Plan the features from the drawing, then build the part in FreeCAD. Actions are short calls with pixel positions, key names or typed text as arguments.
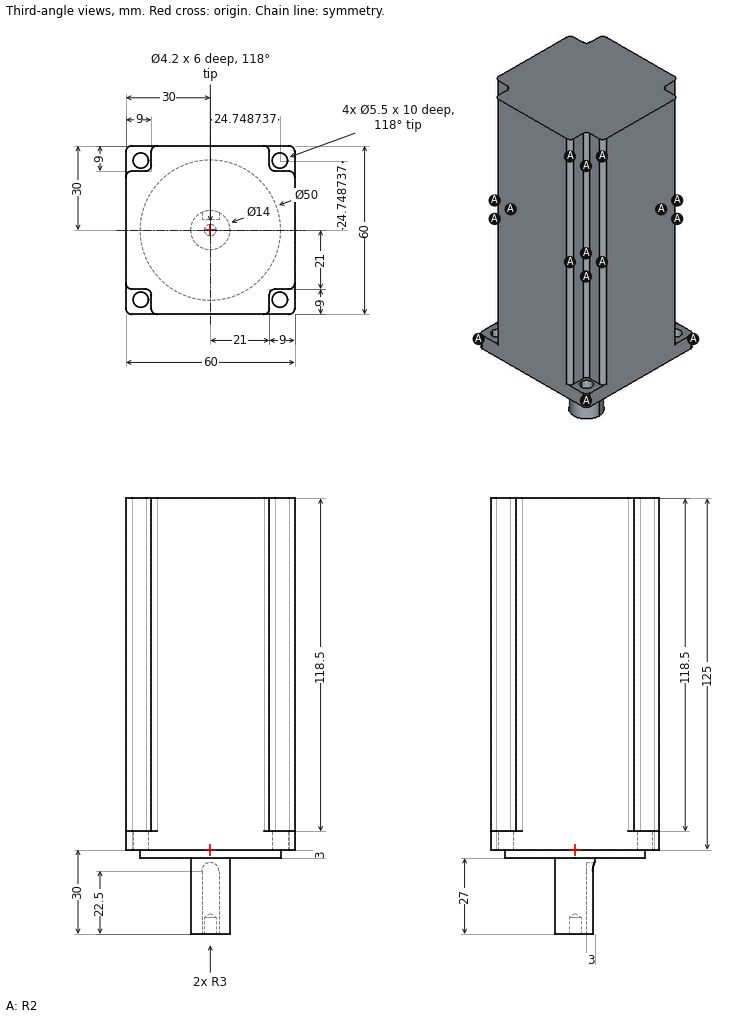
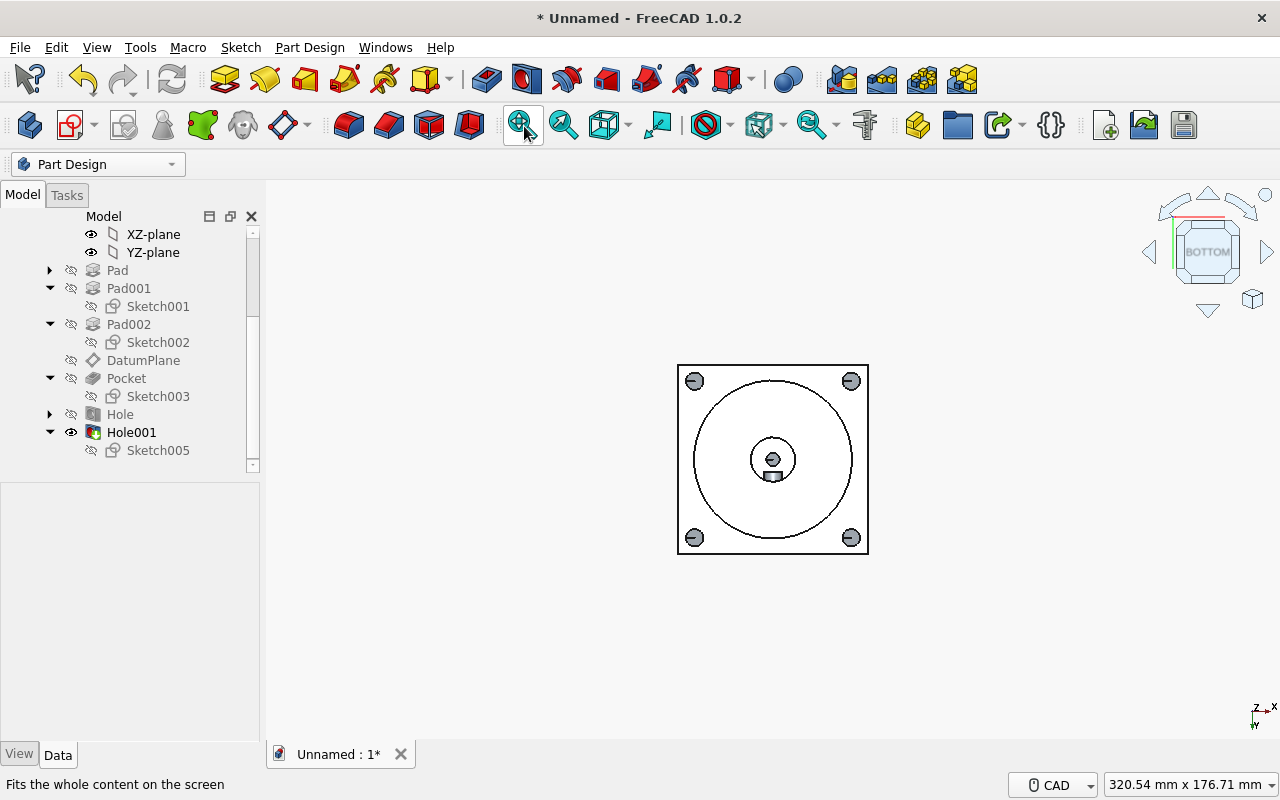
key(0)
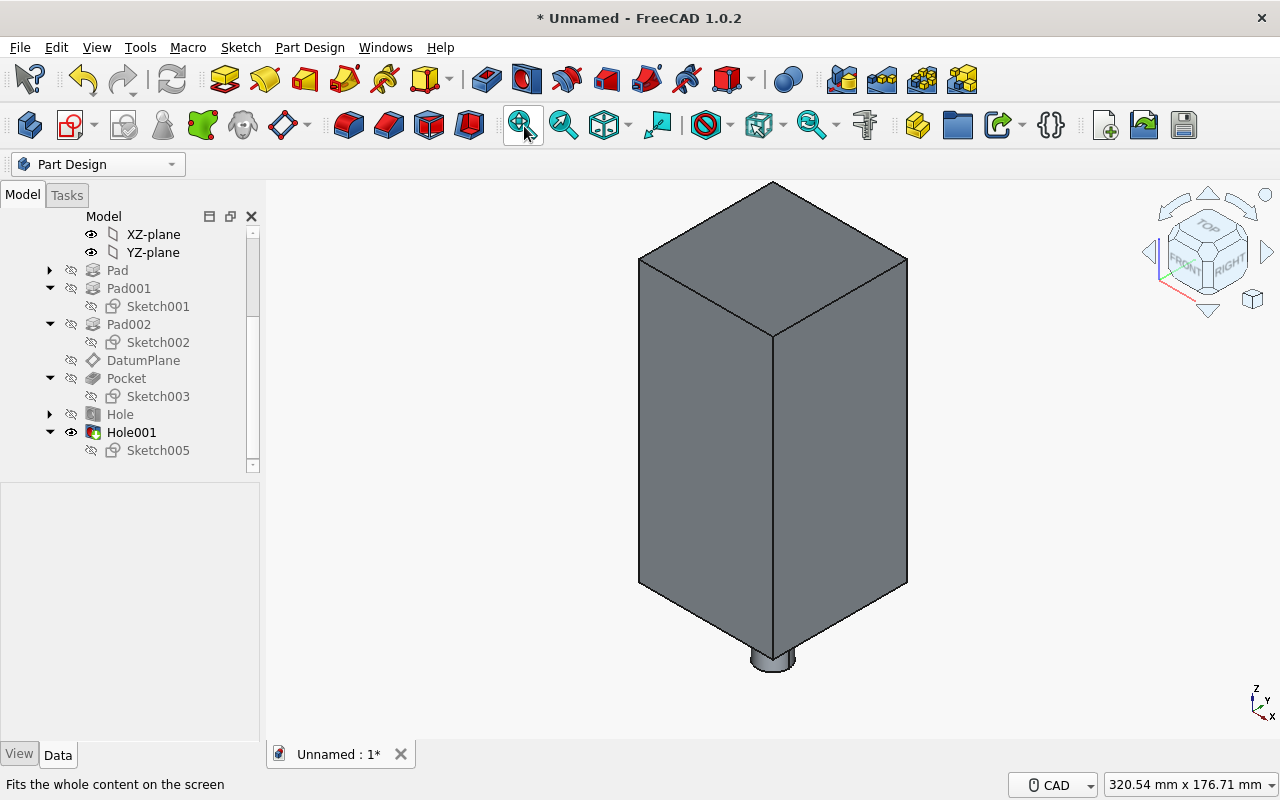
click(773, 258)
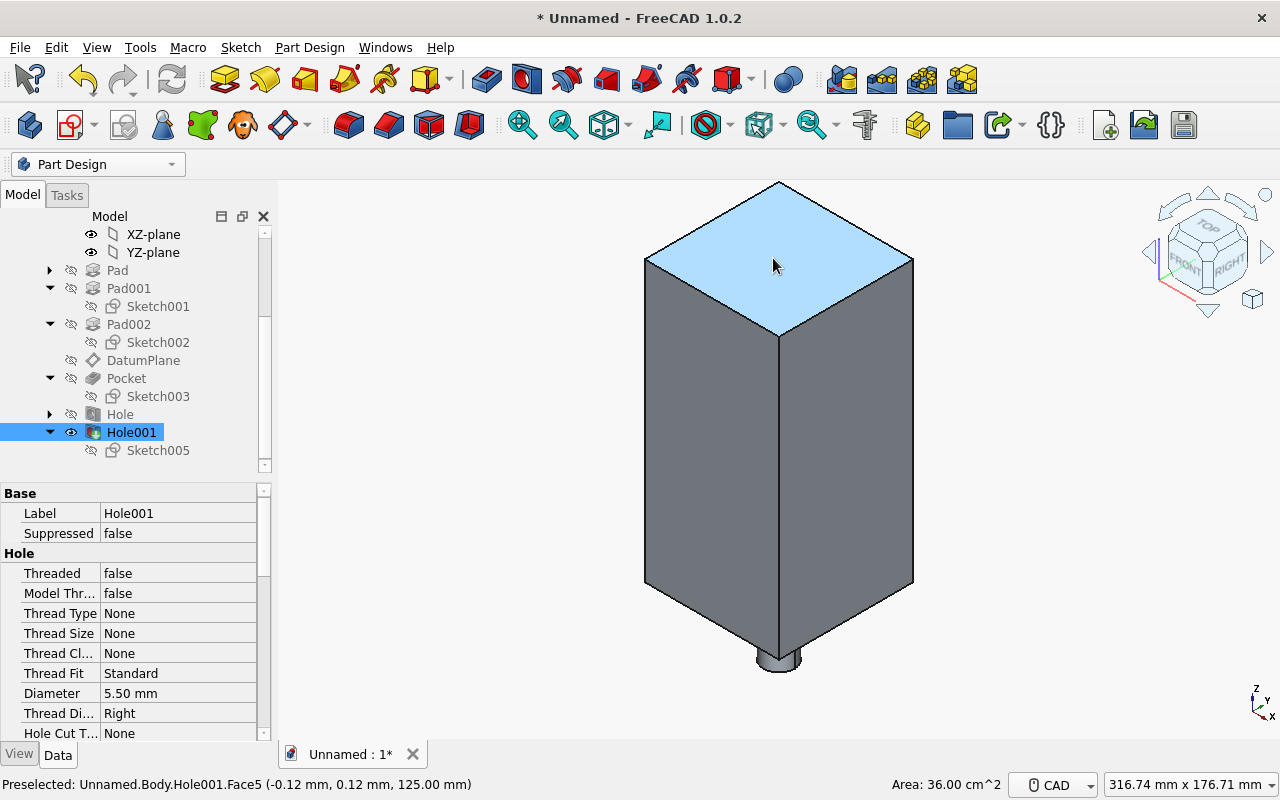
click(70, 126)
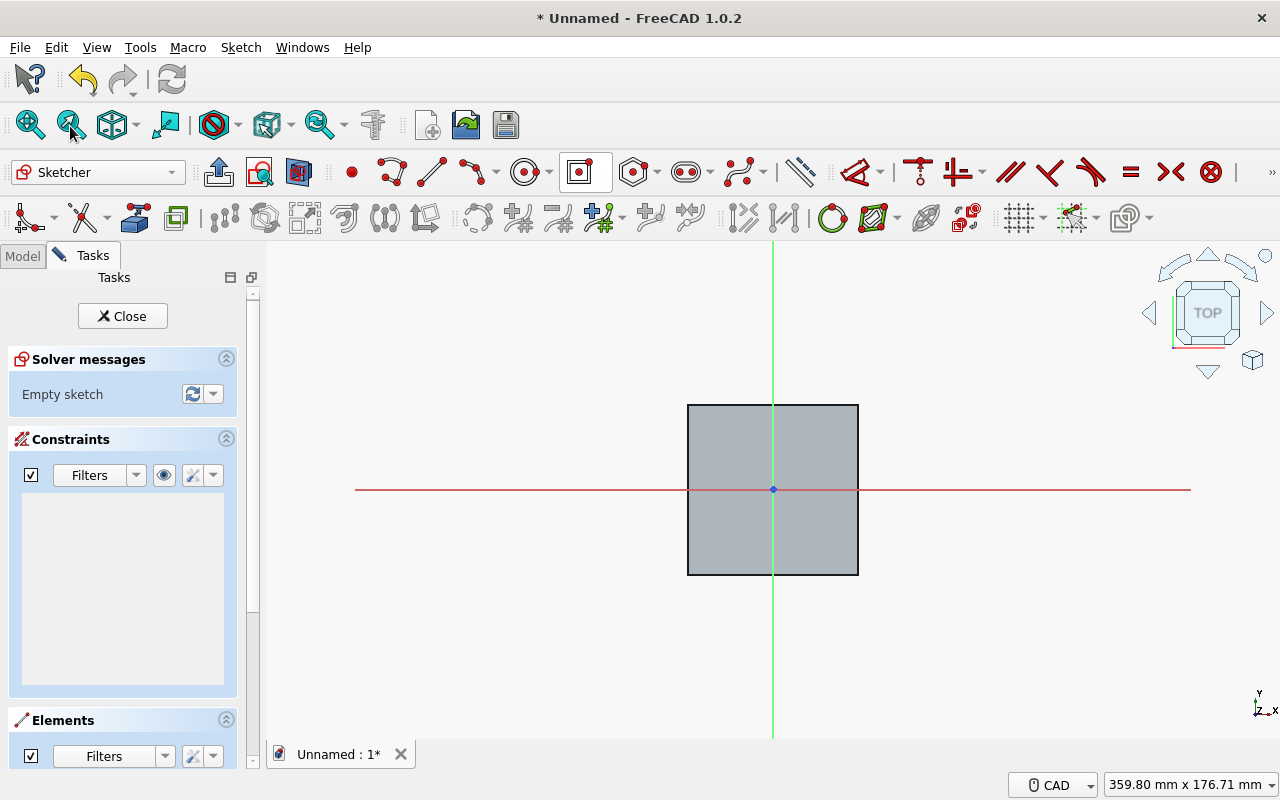
scroll(701, 412, up, 13)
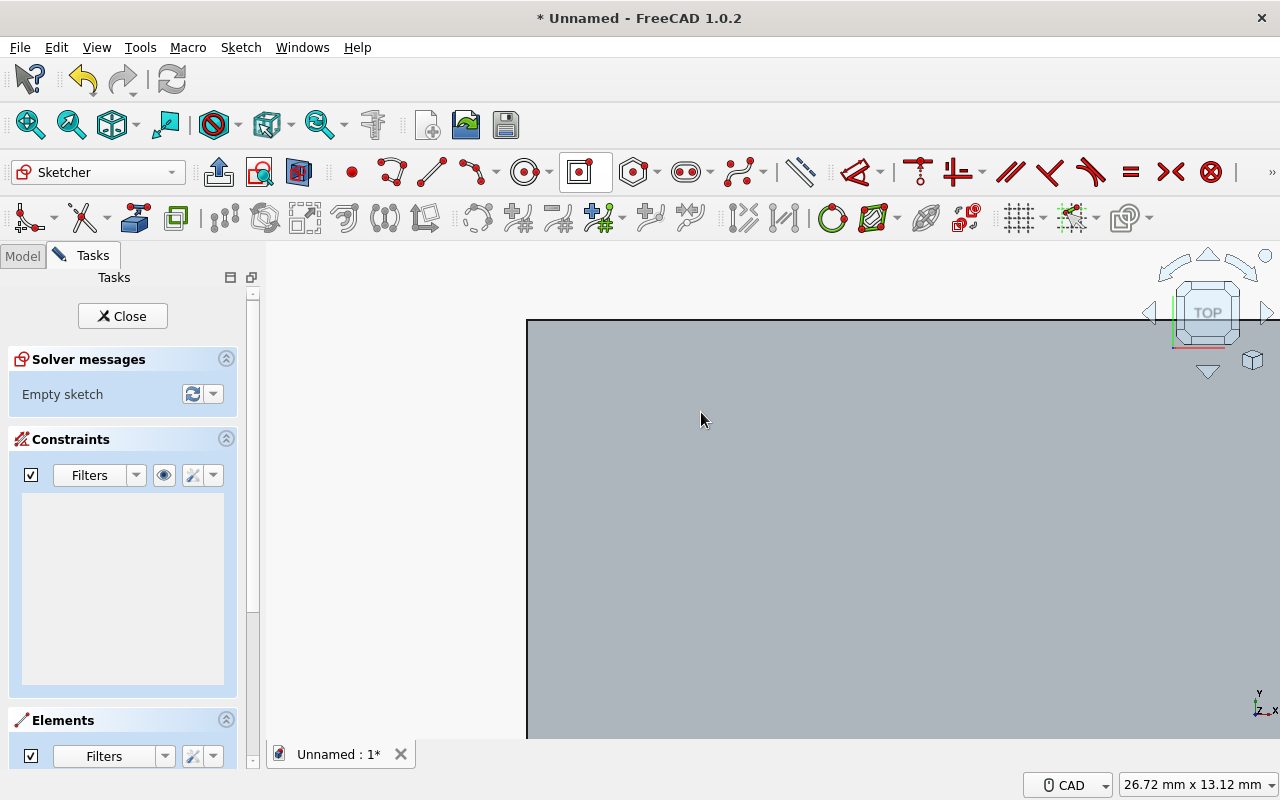
click(606, 172)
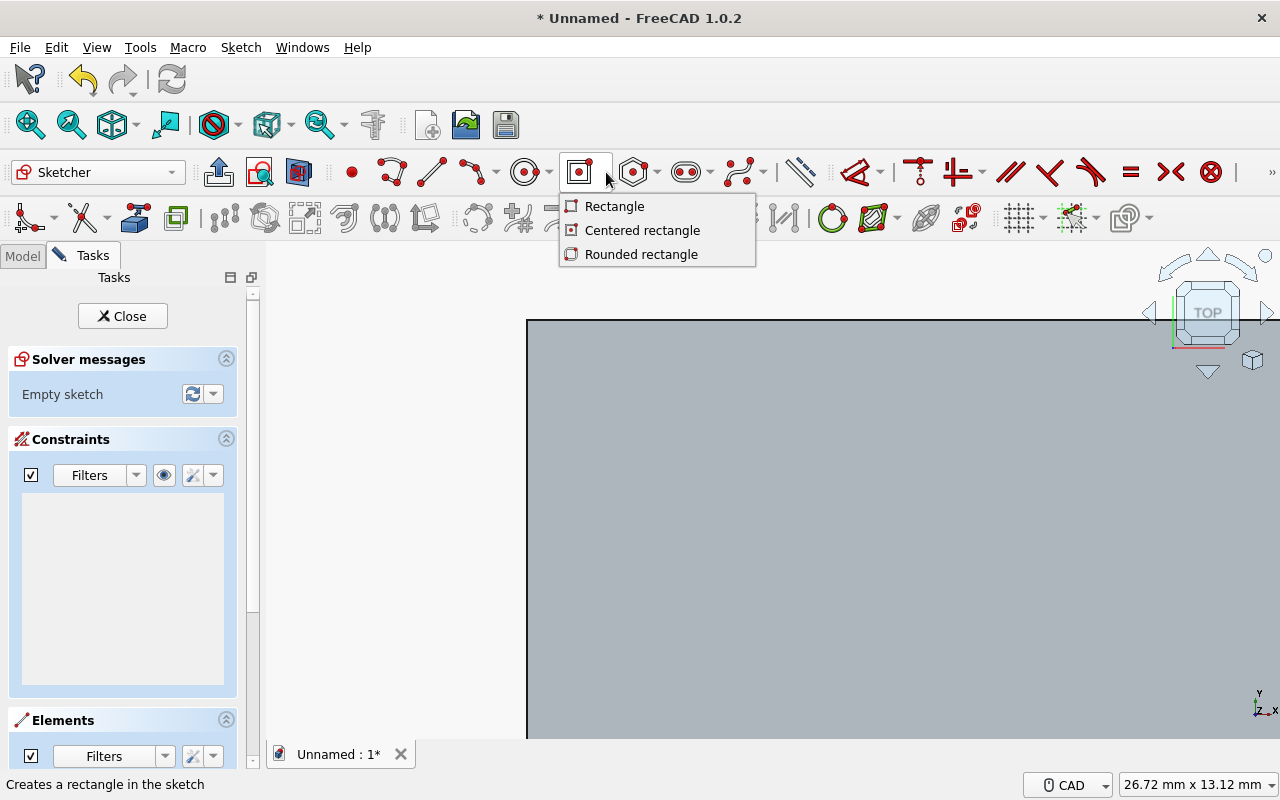
click(658, 206)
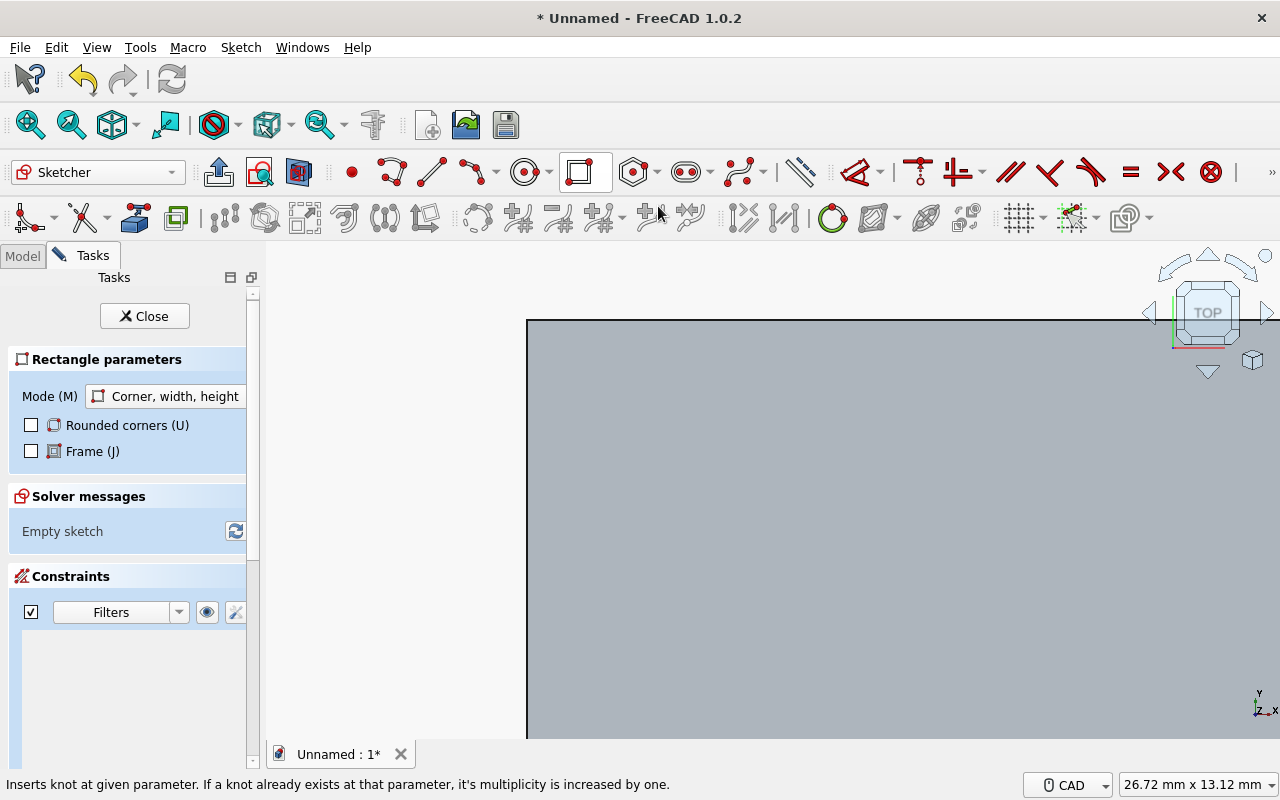
click(527, 320)
move(868, 661)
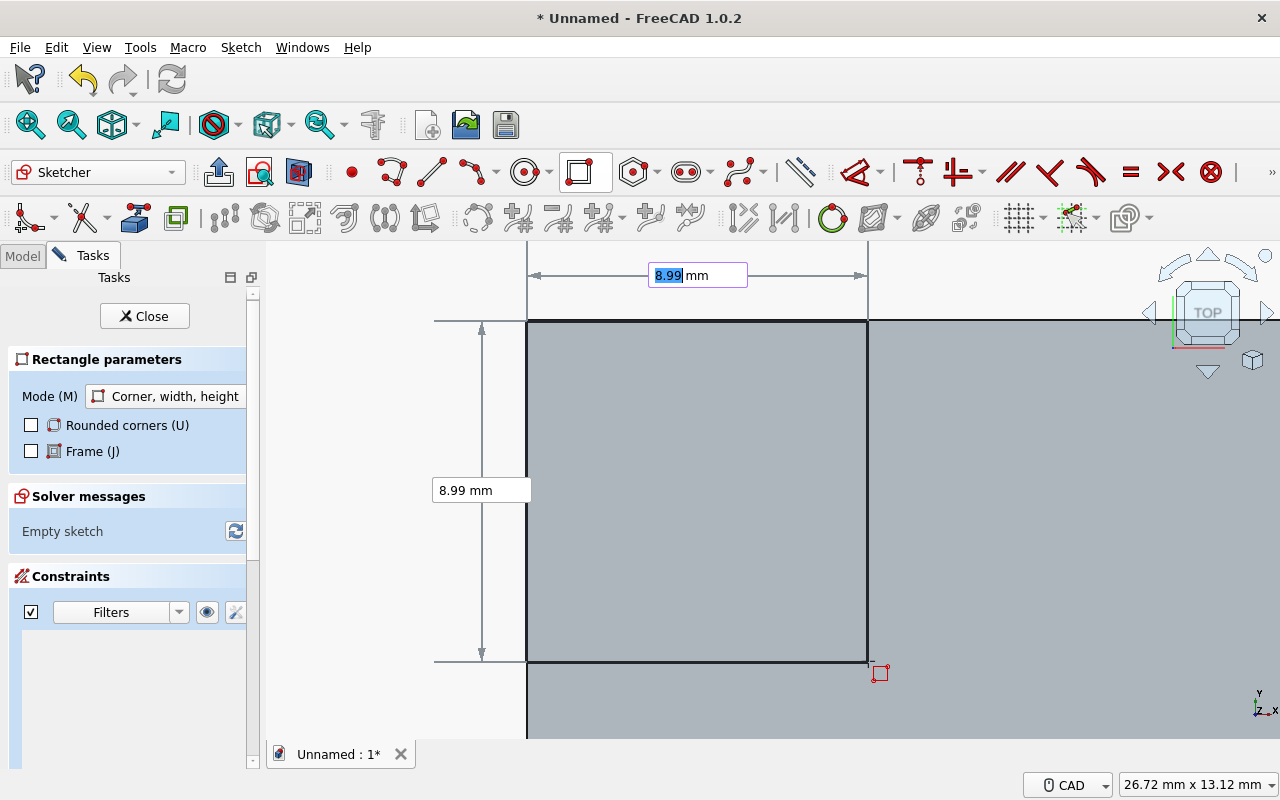
text(9)
key(Tab)
text(9)
key(Return)
key(Escape)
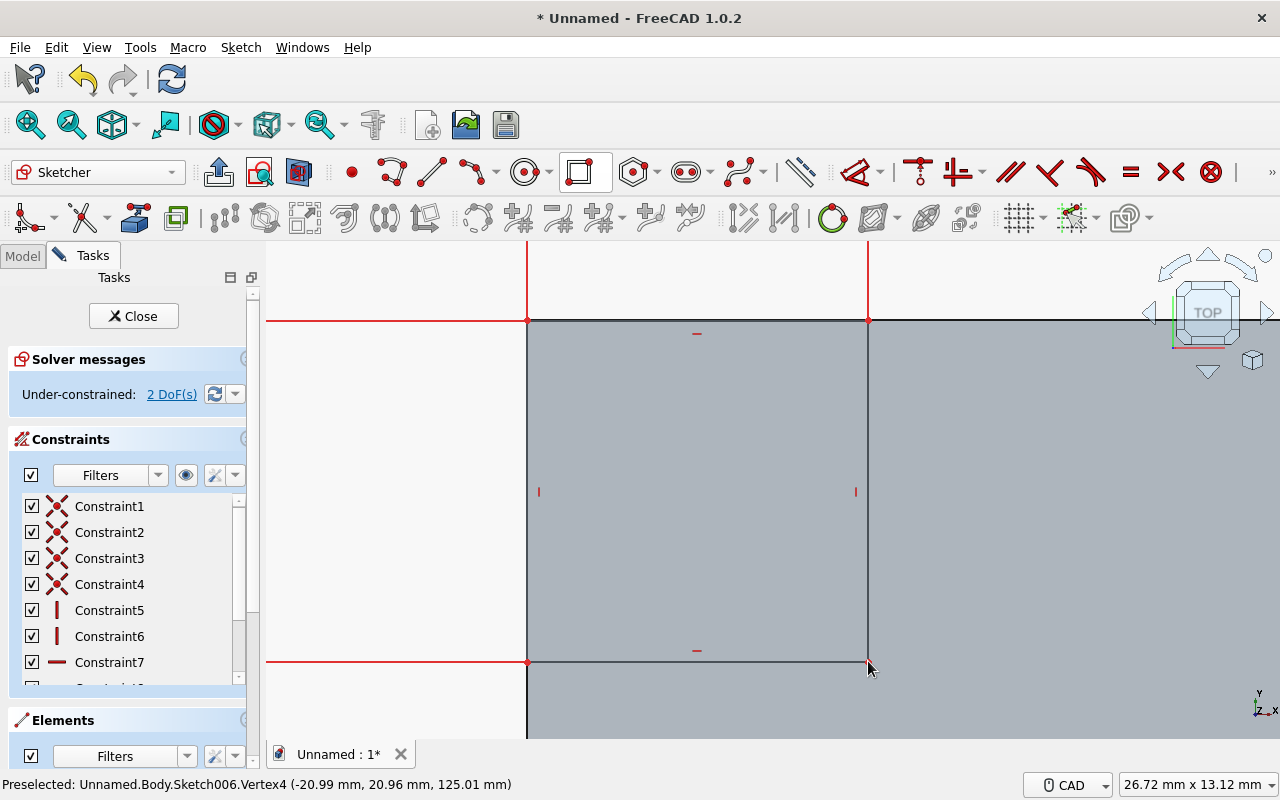
click(856, 172)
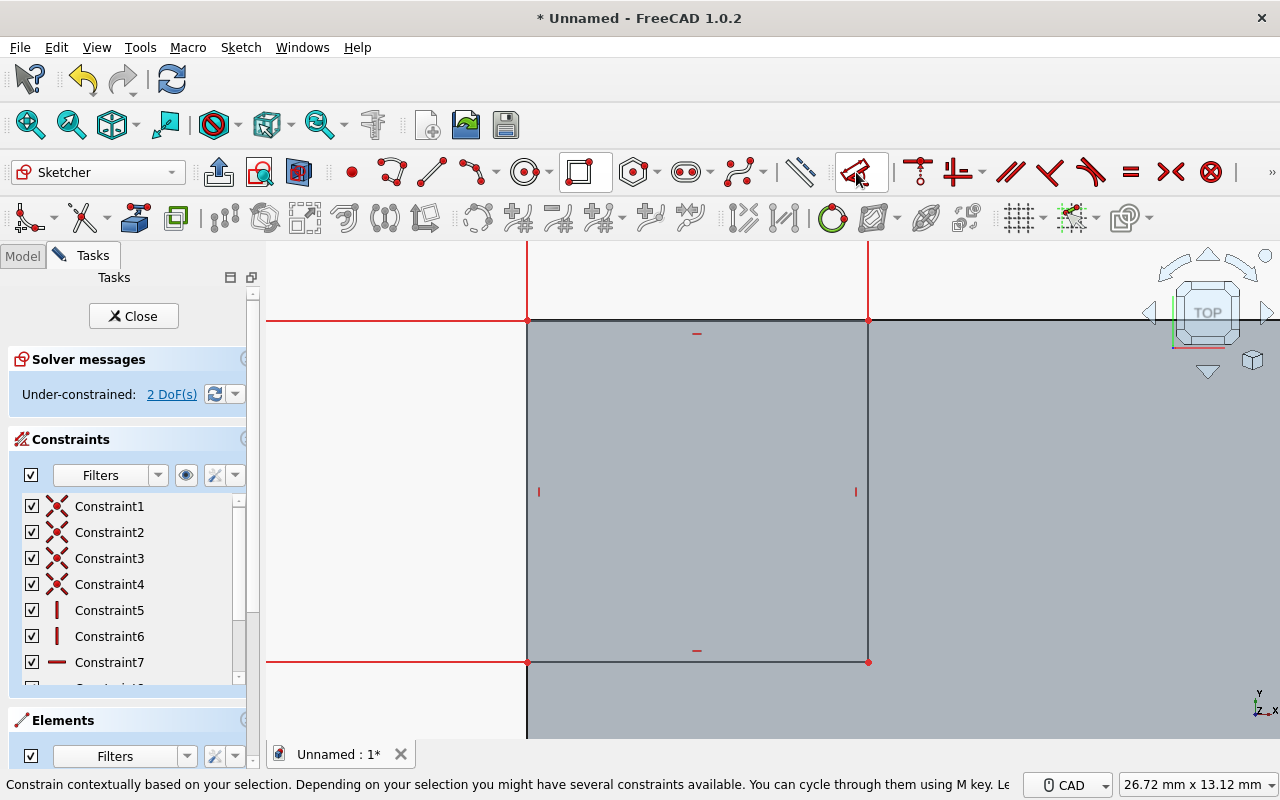
click(527, 321)
click(821, 287)